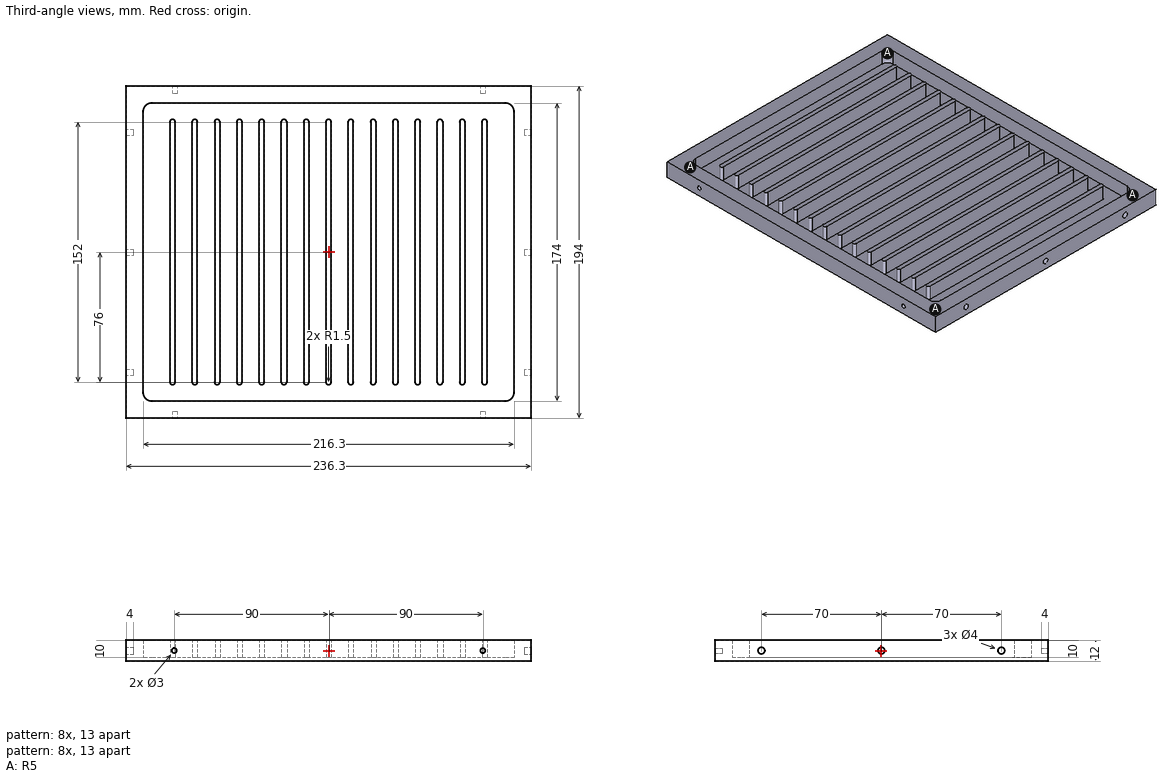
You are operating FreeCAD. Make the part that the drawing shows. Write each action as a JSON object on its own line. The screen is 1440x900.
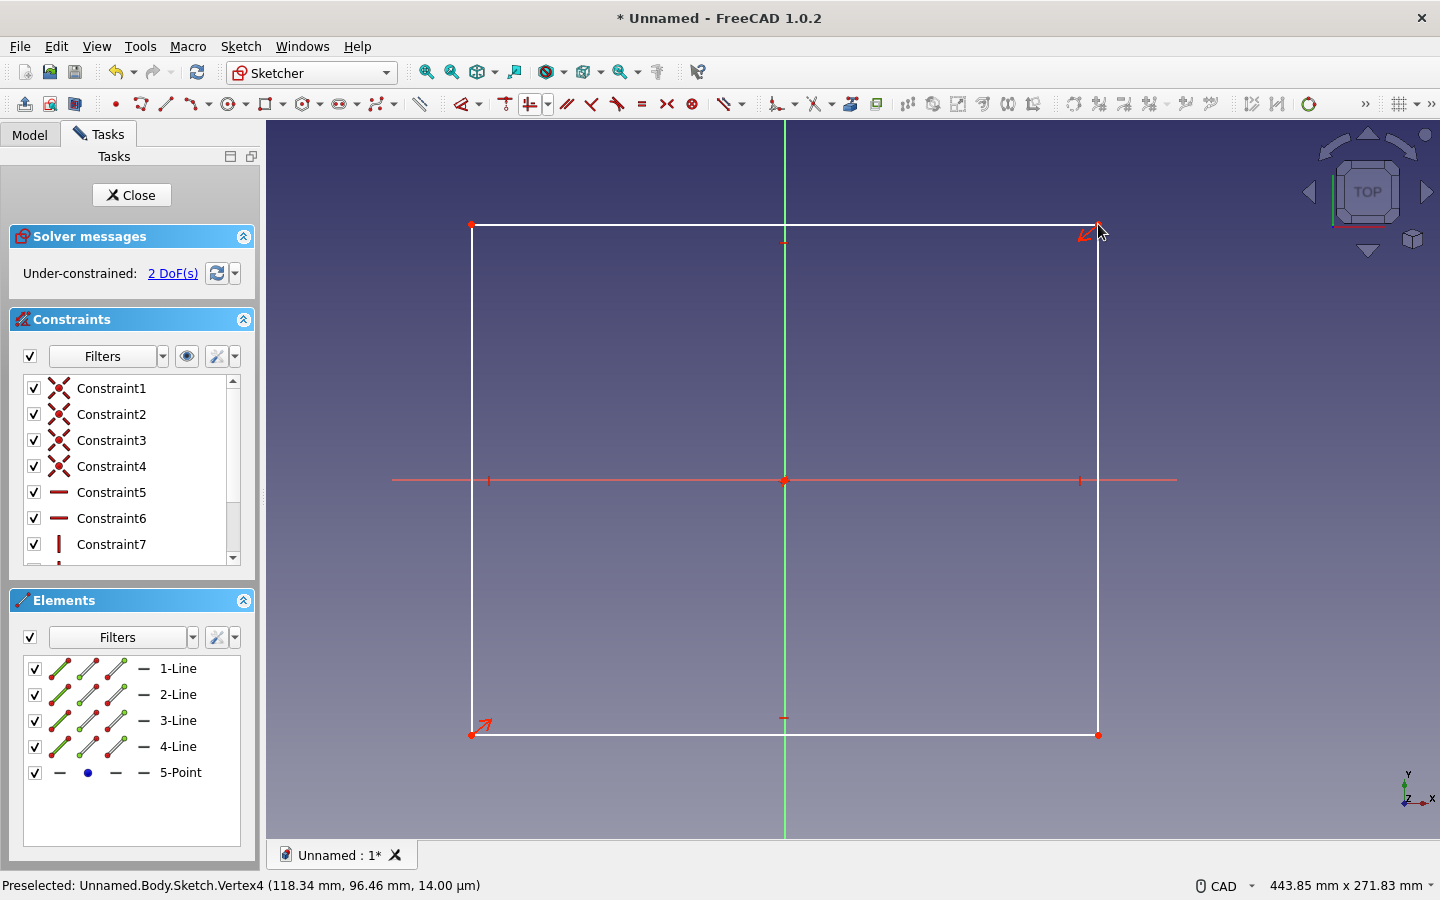
{"action": "left_click", "coordinate": [460, 104]}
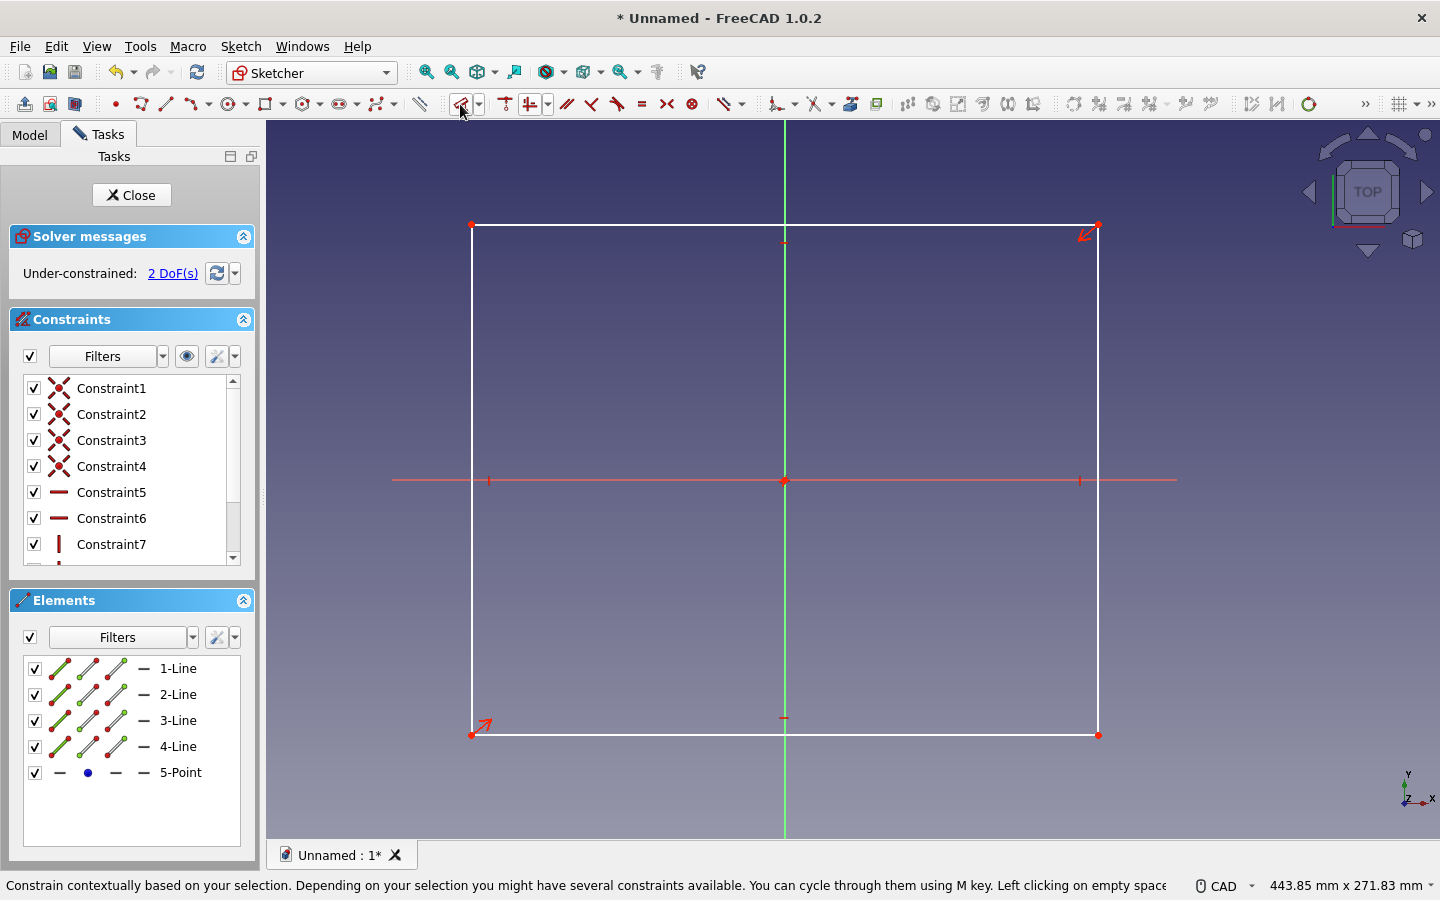
{"action": "left_click", "coordinate": [1098, 582]}
{"action": "left_click", "coordinate": [1132, 363]}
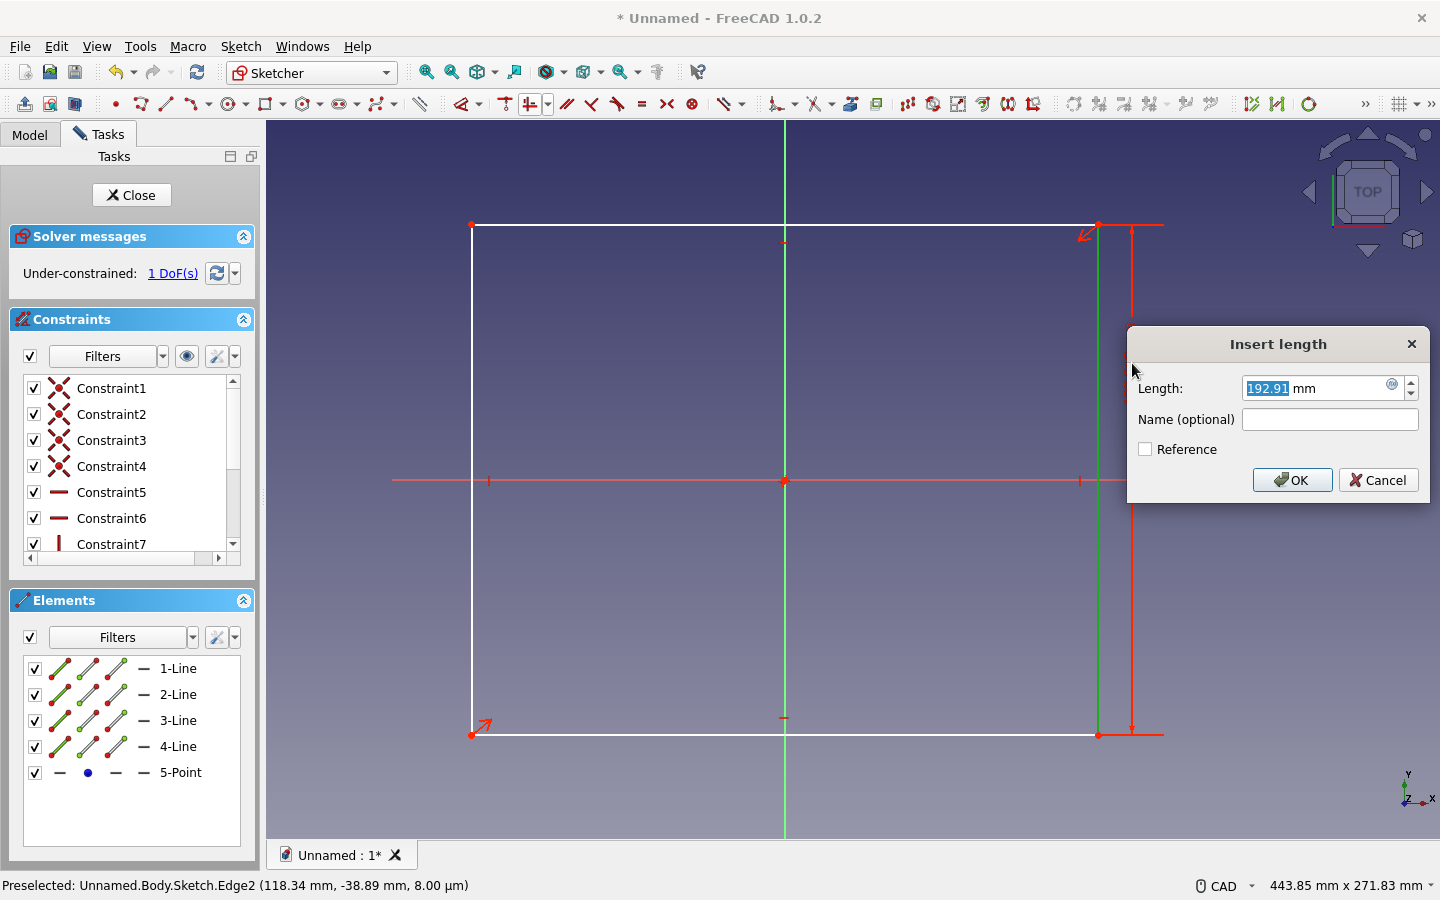
{"action": "type", "text": "194"}
{"action": "key", "text": "Return"}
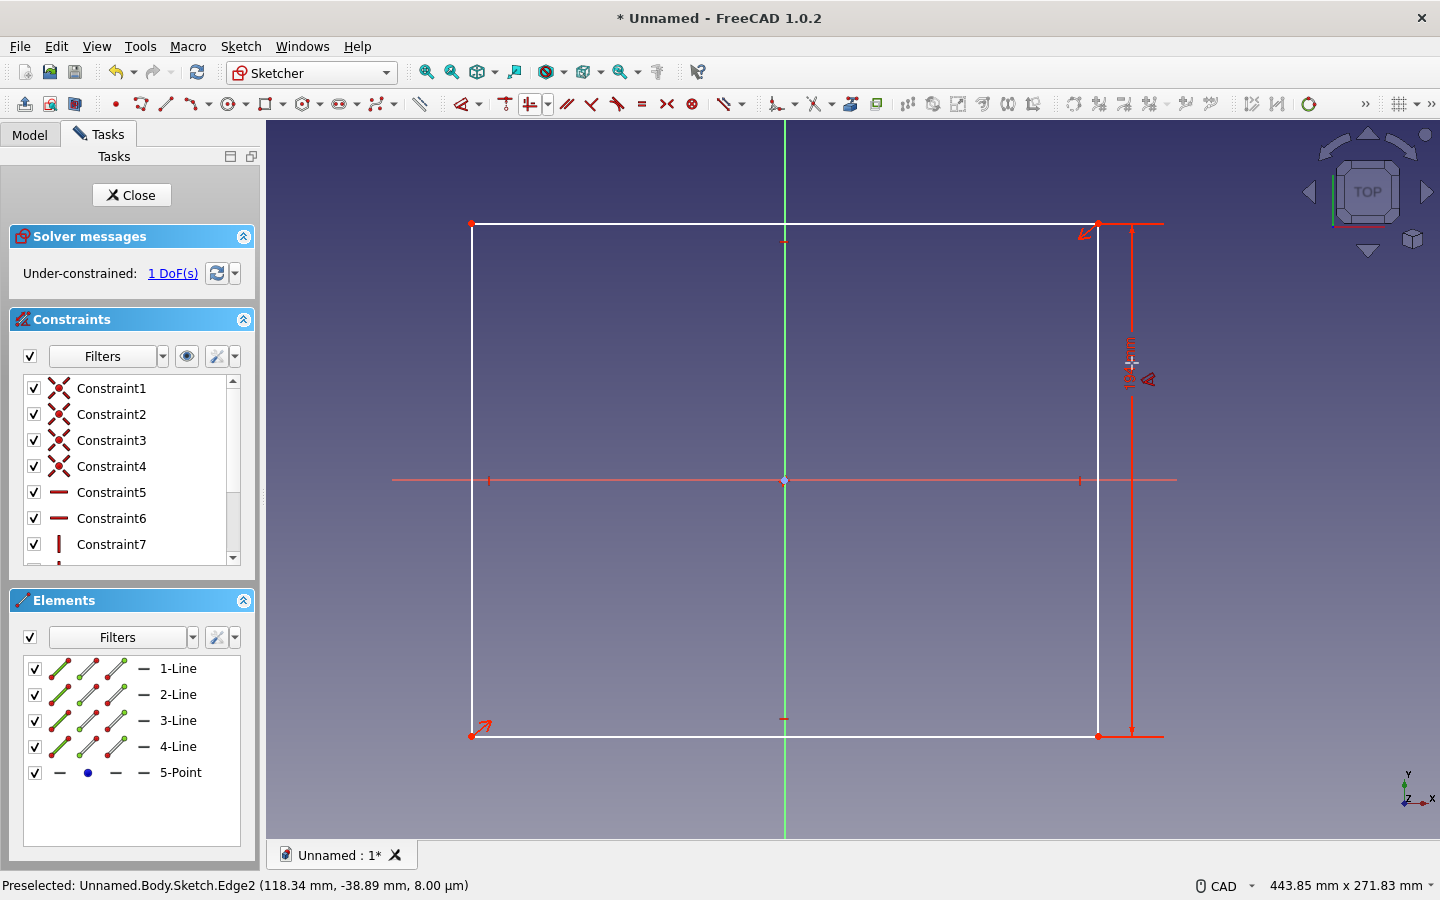
{"action": "left_click", "coordinate": [660, 737]}
{"action": "left_click", "coordinate": [641, 771]}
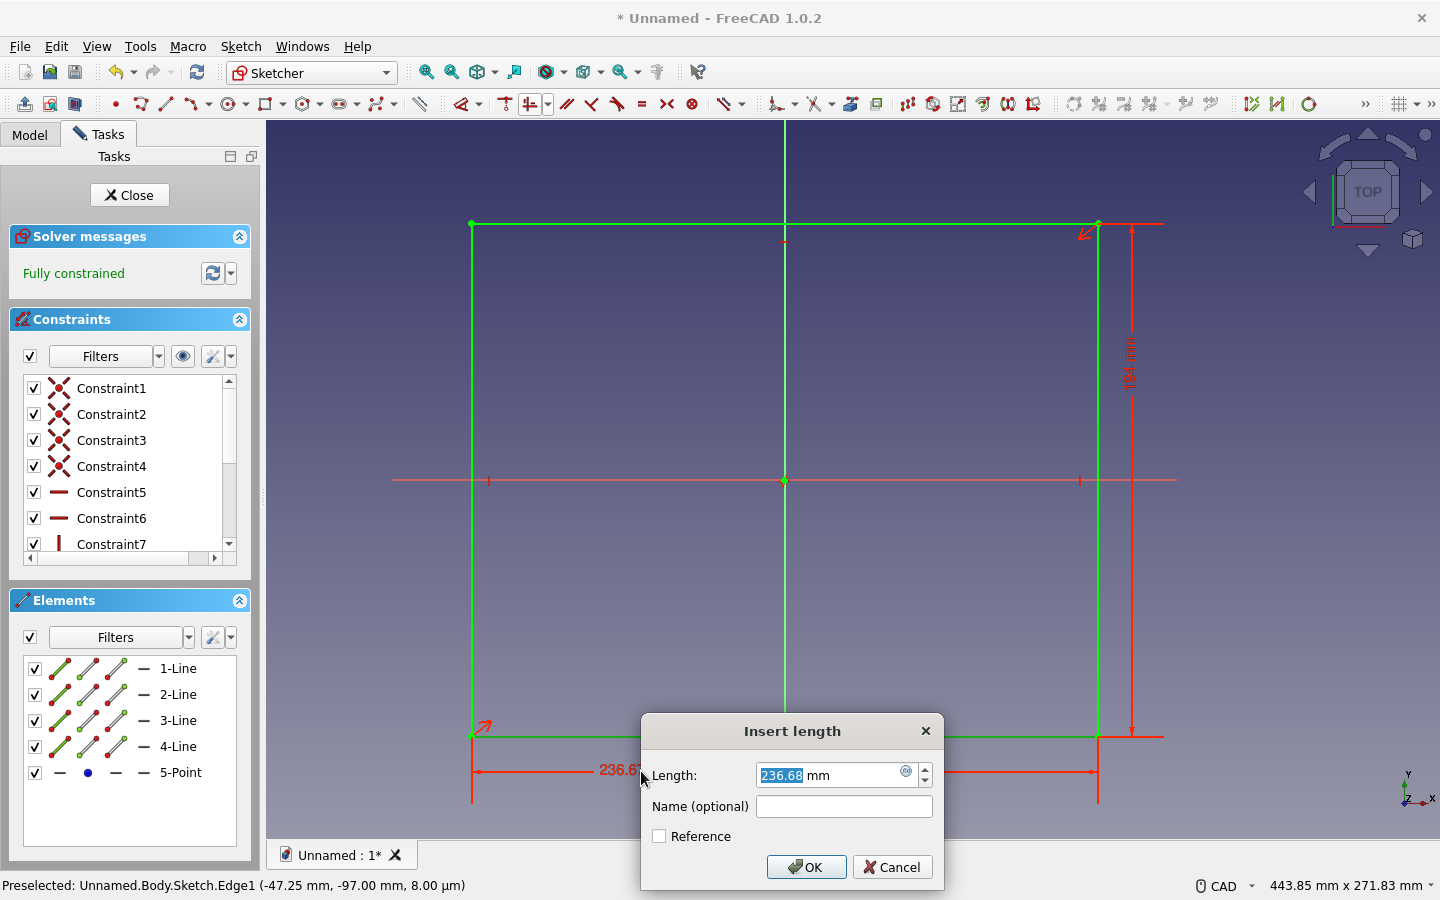
{"action": "type", "text": "236.3"}
{"action": "key", "text": "Return"}
{"action": "key", "text": "Escape"}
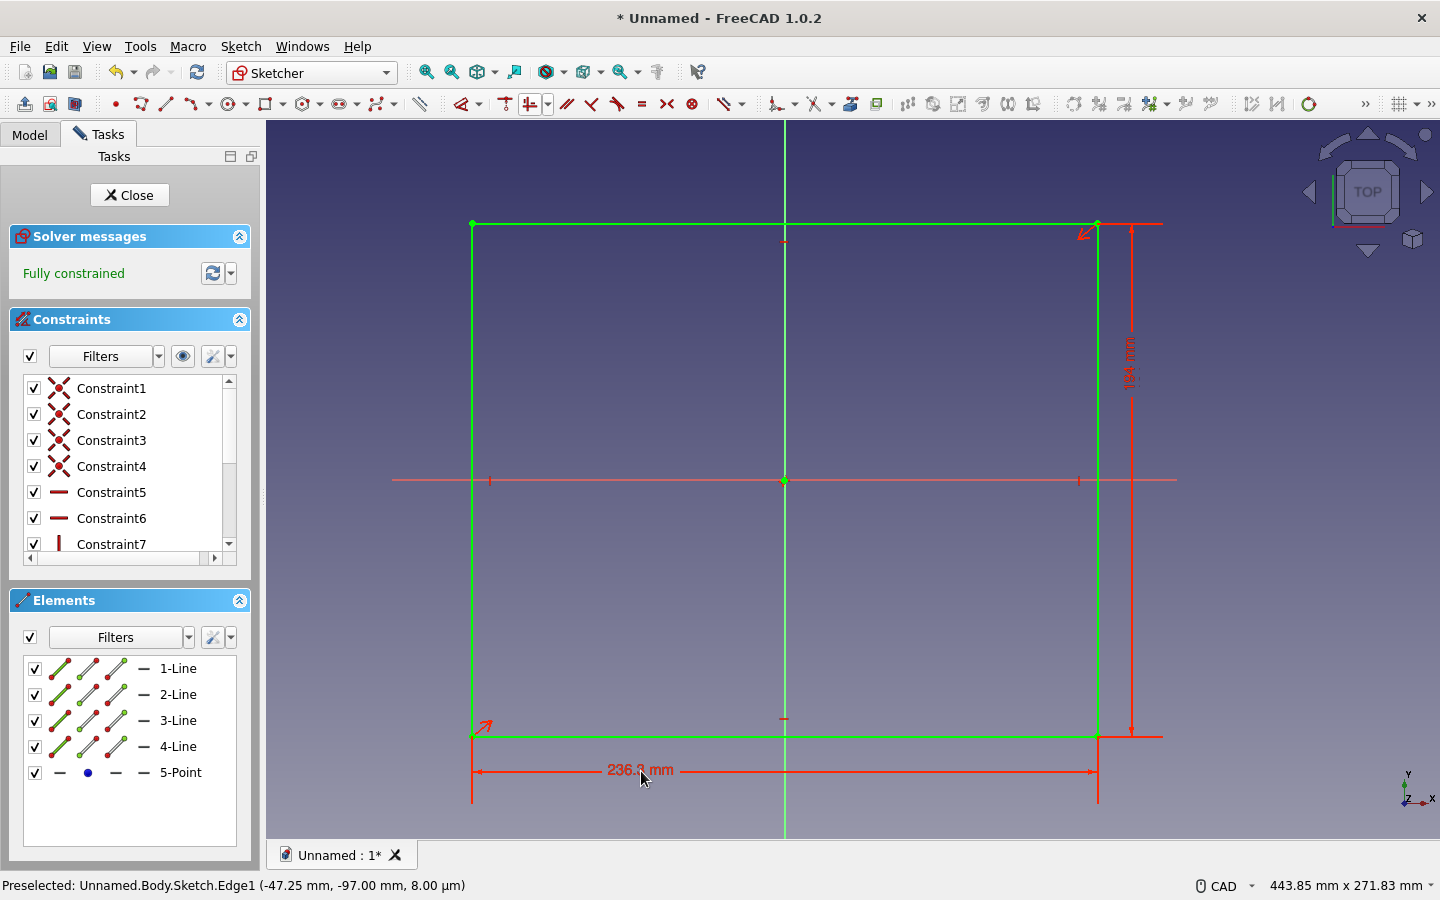
{"action": "left_click", "coordinate": [130, 195]}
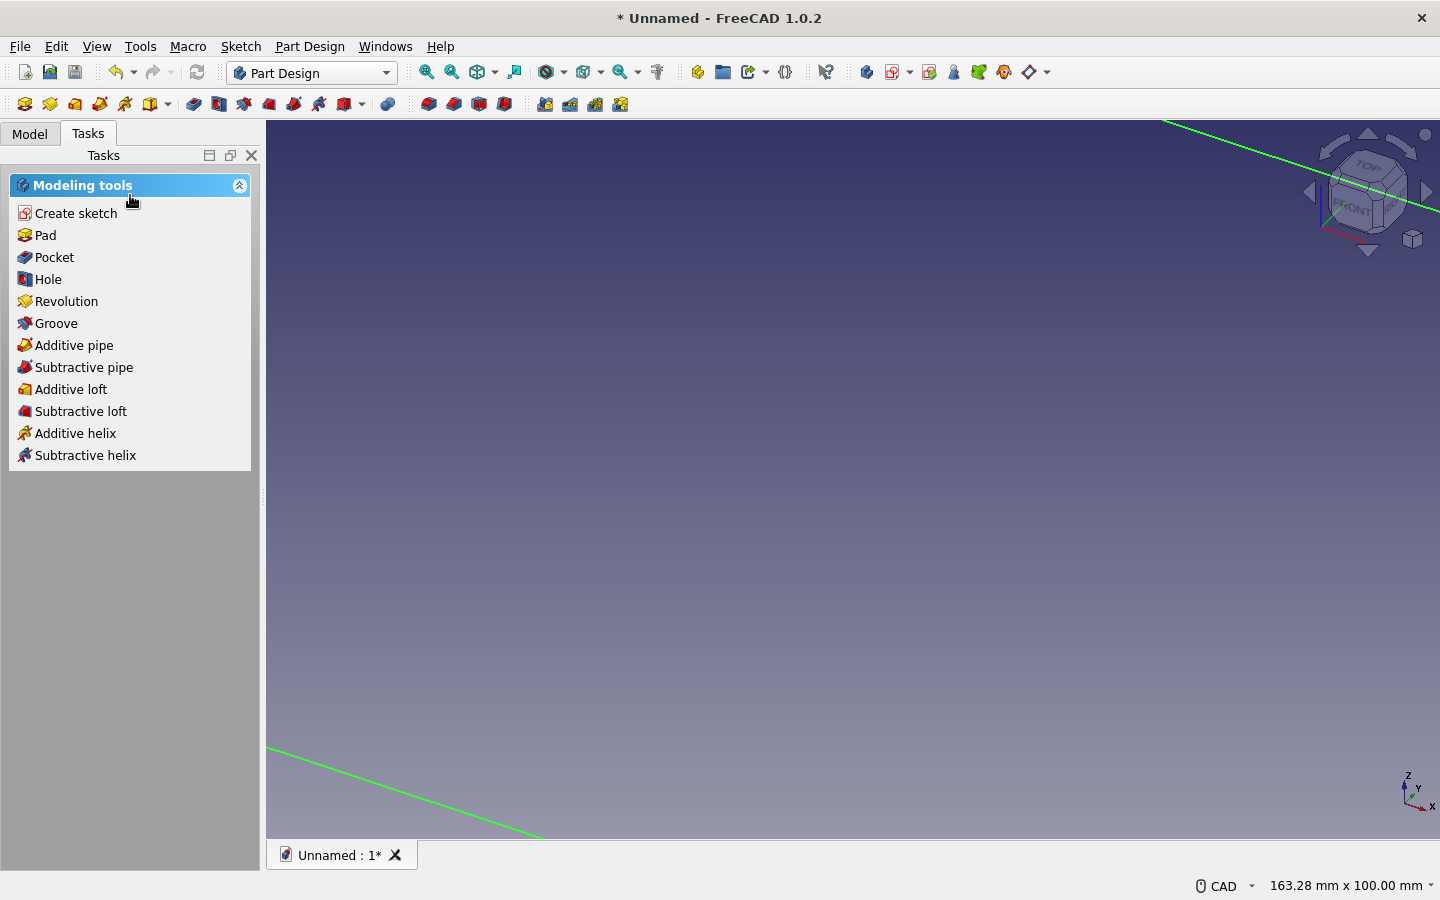
{"action": "left_click", "coordinate": [25, 104]}